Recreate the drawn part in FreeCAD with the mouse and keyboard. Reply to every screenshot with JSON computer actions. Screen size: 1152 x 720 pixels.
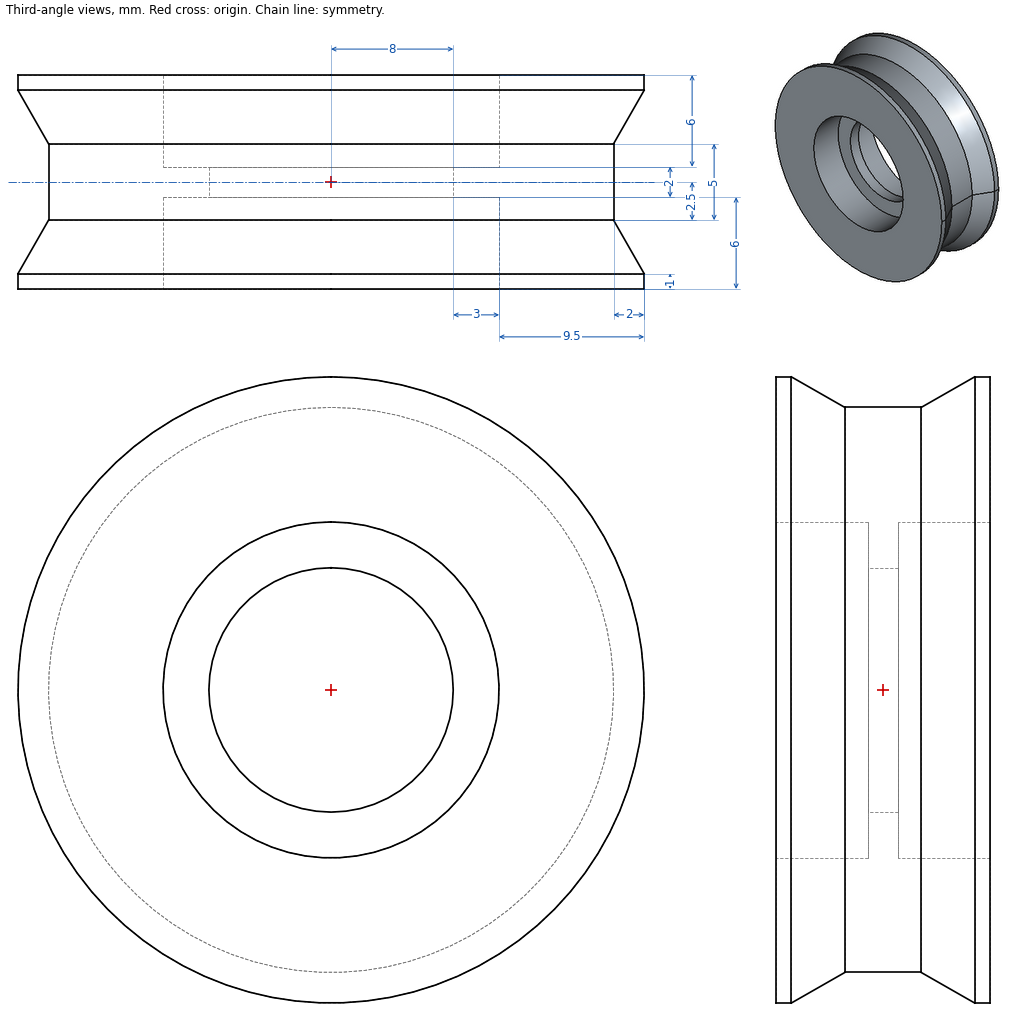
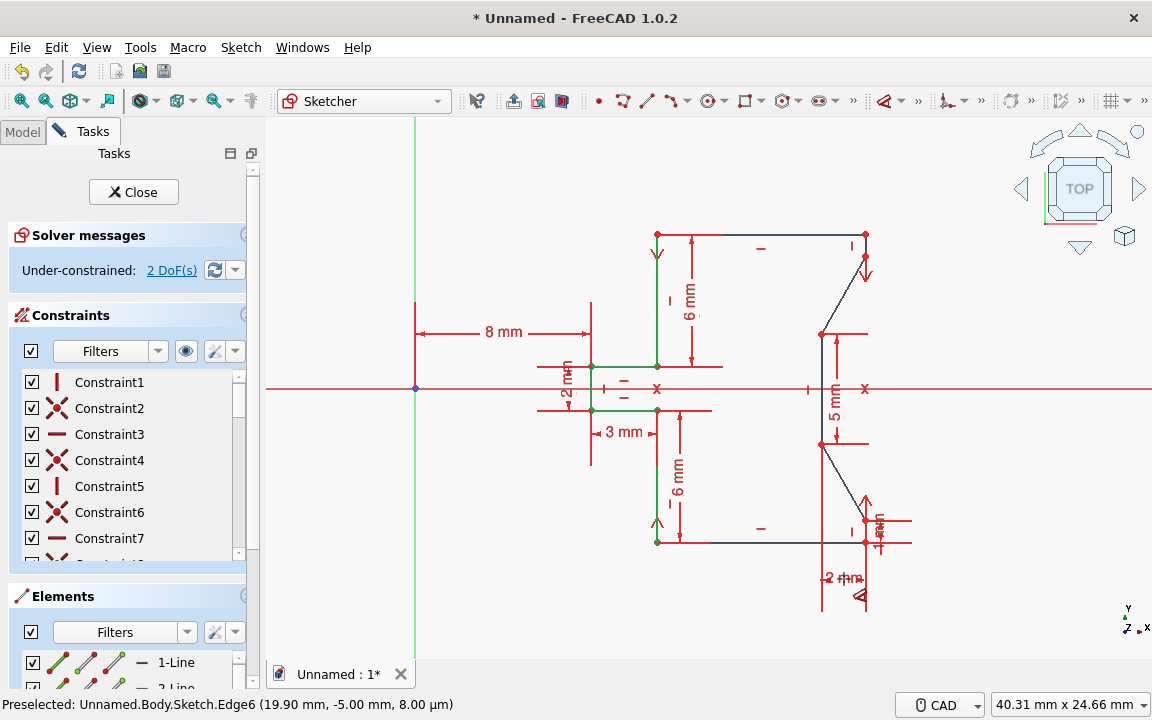
{"action": "left_click", "coordinate": [720, 543]}
{"action": "left_click", "coordinate": [761, 577]}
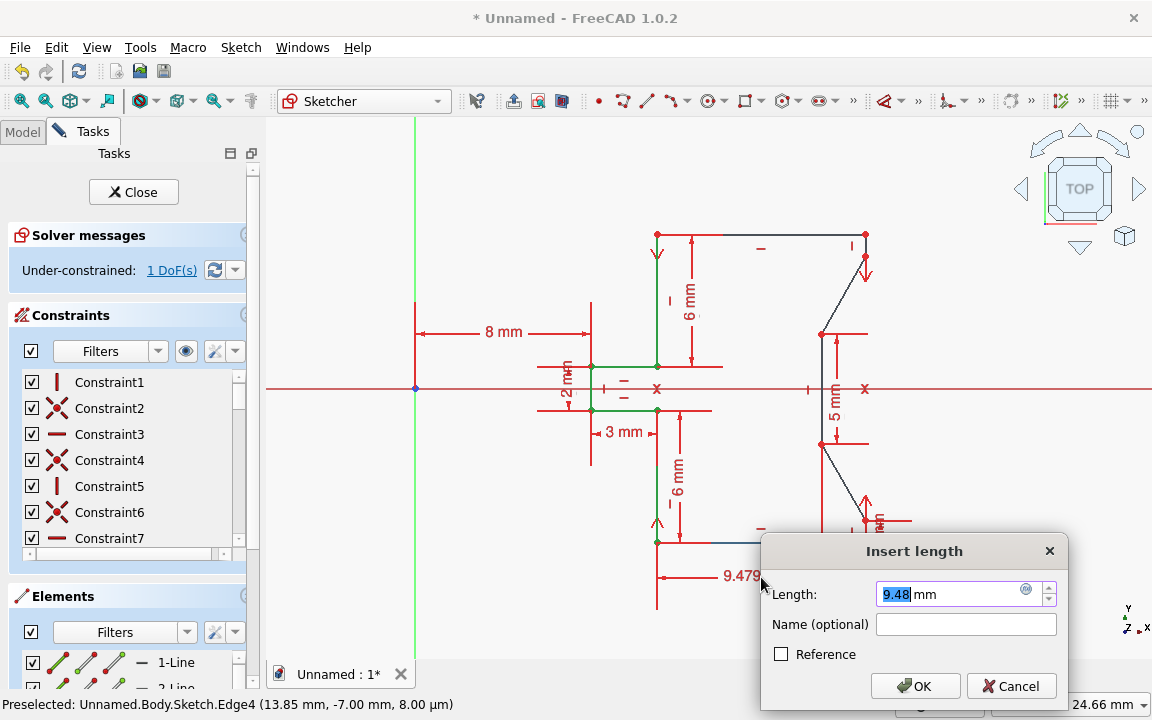
{"action": "type", "text": "9.5"}
{"action": "key", "text": "Return"}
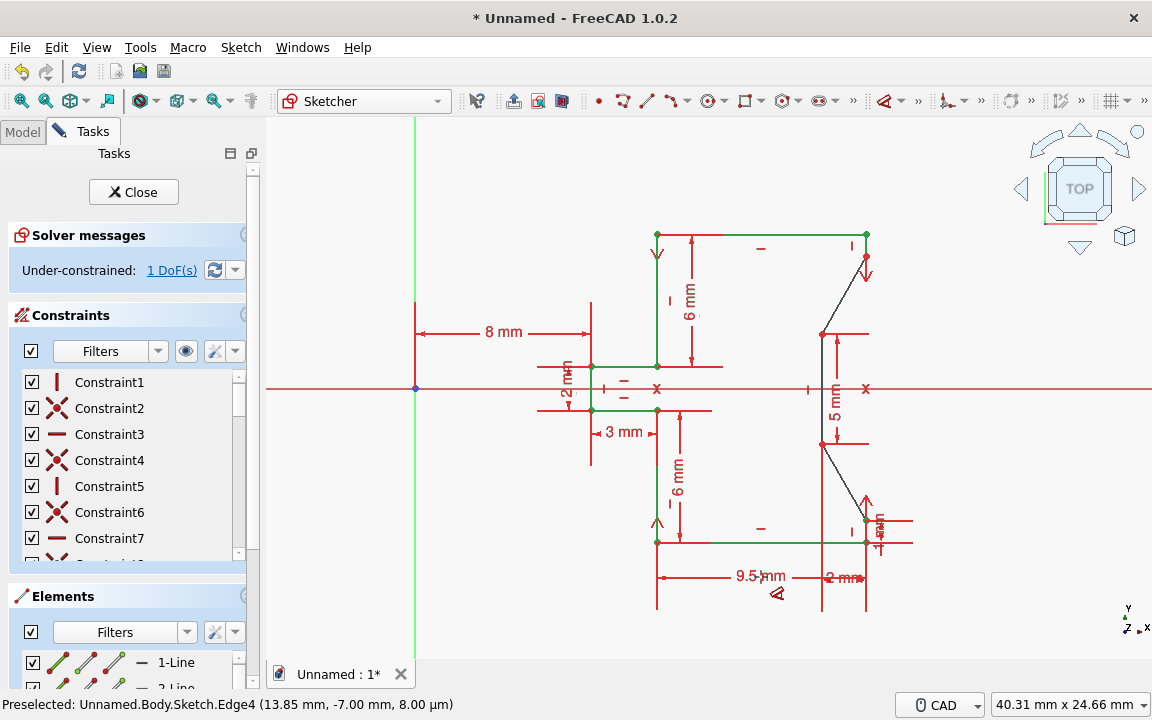
{"action": "left_click", "coordinate": [822, 444]}
{"action": "left_click", "coordinate": [381, 416]}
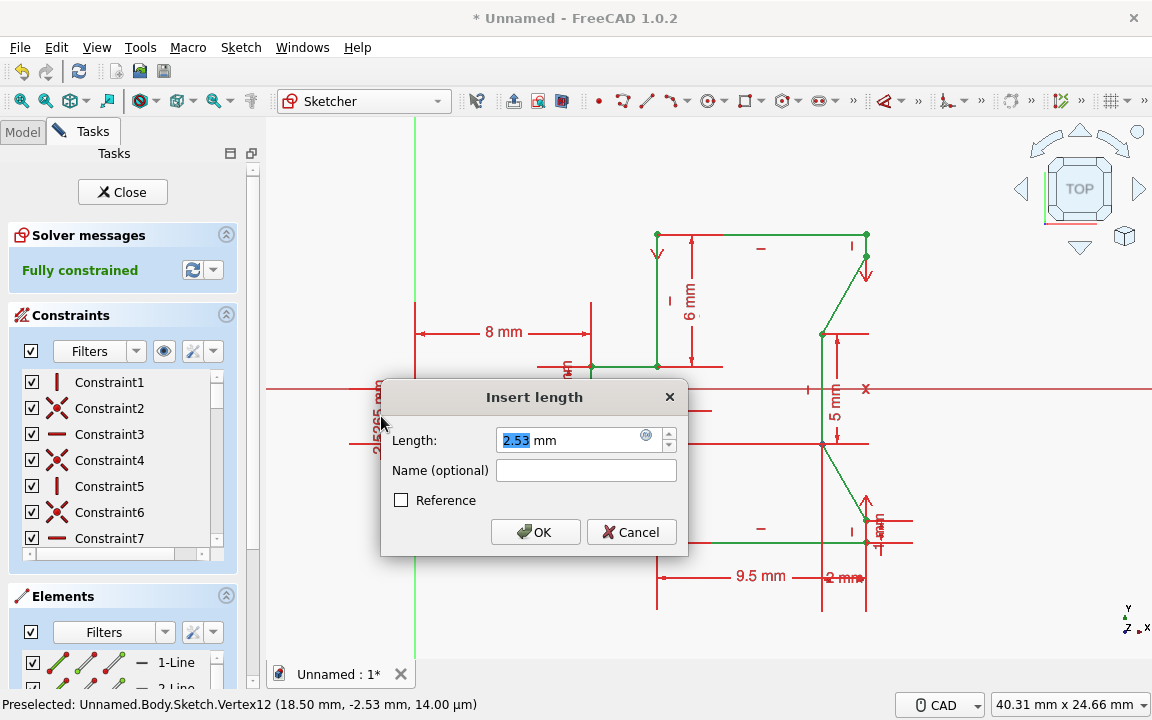
{"action": "type", "text": "2.5"}
{"action": "key", "text": "Return"}
{"action": "key", "text": "Escape"}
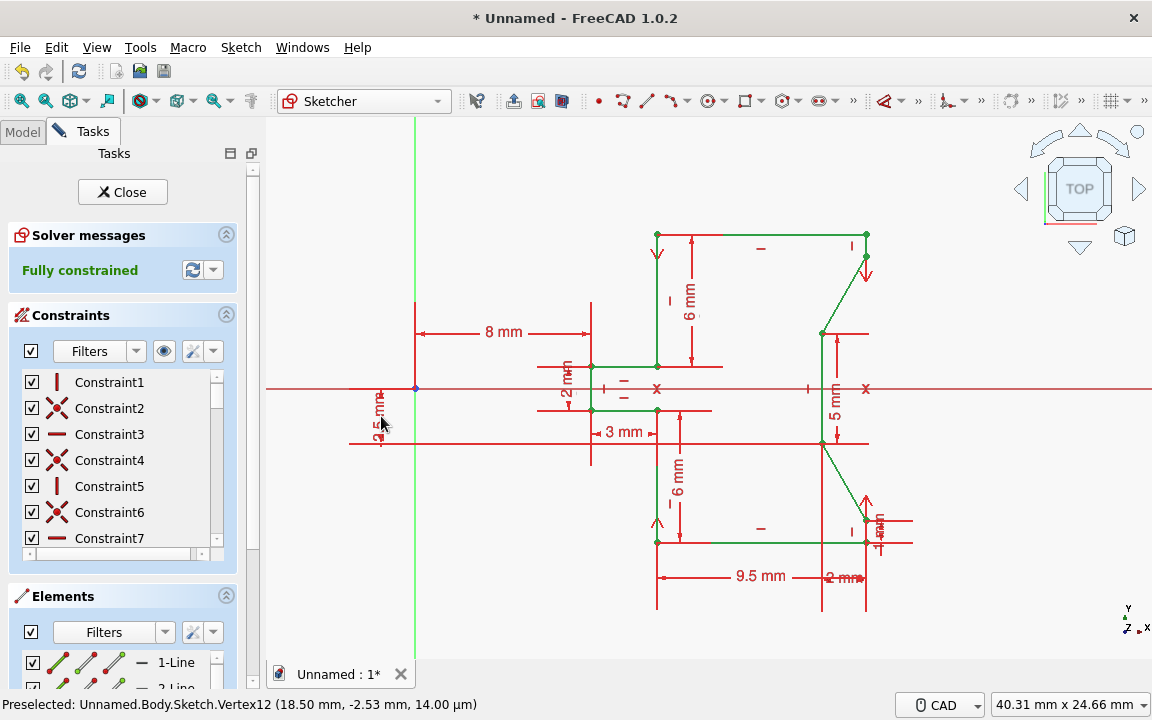
{"action": "left_click", "coordinate": [123, 192]}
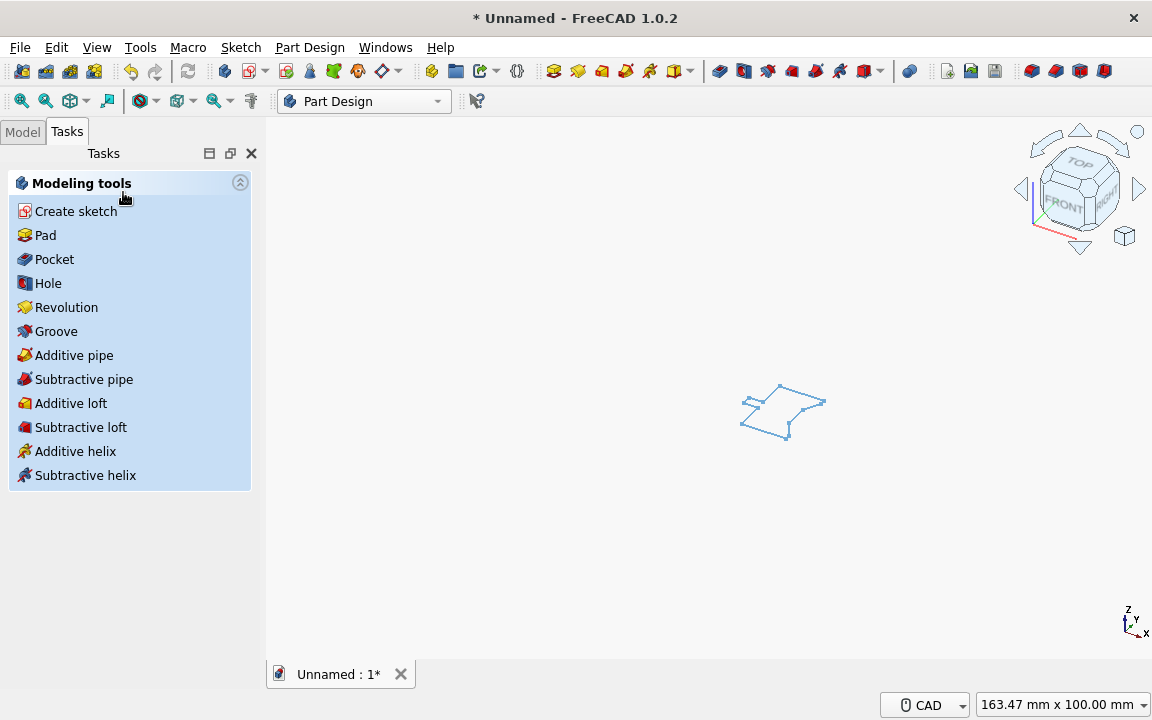
{"action": "left_click", "coordinate": [578, 72]}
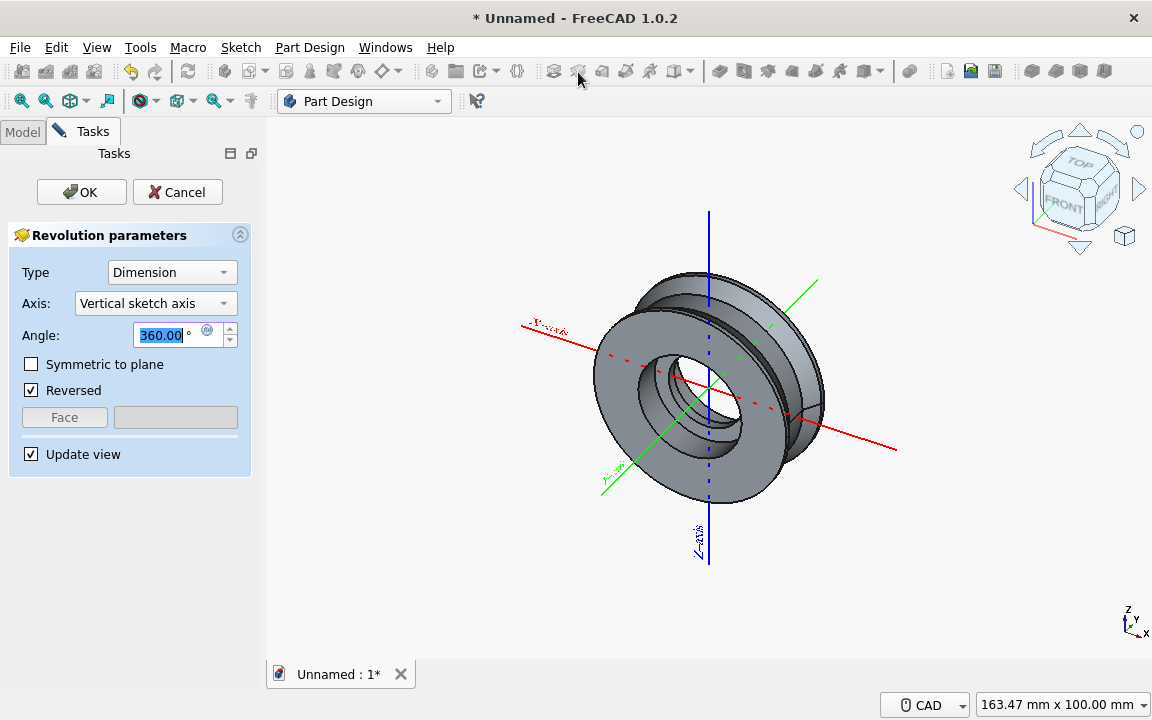
{"action": "left_click", "coordinate": [82, 192]}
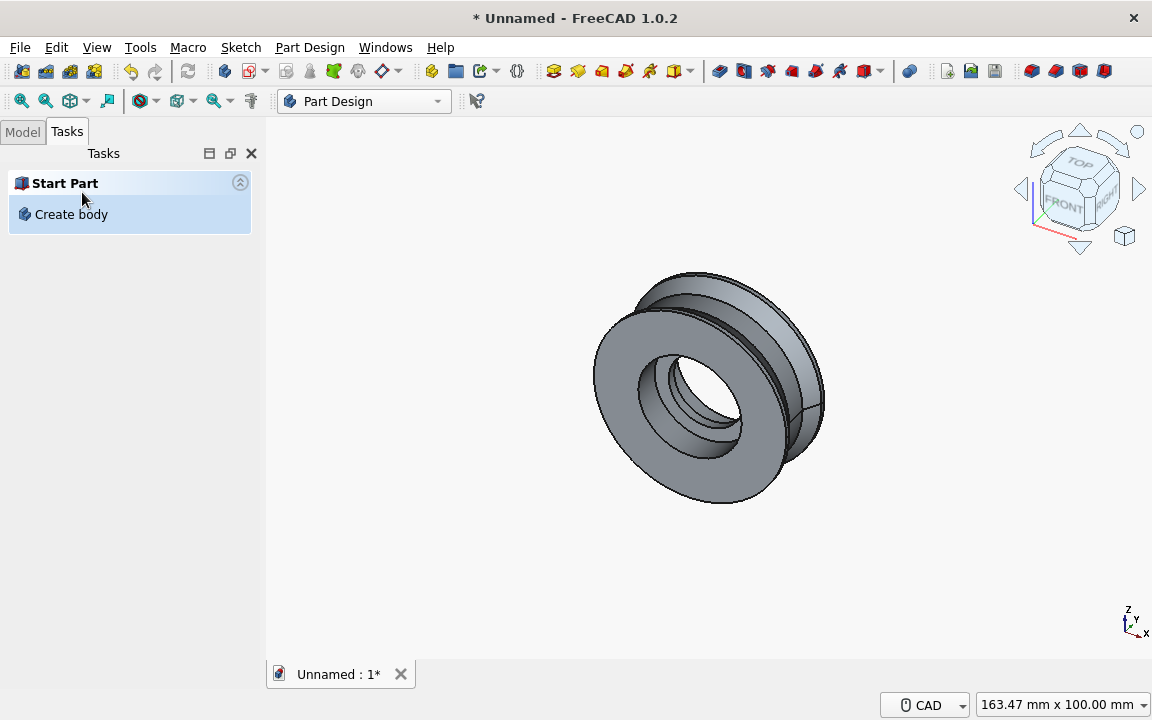
{"action": "key", "text": "0"}